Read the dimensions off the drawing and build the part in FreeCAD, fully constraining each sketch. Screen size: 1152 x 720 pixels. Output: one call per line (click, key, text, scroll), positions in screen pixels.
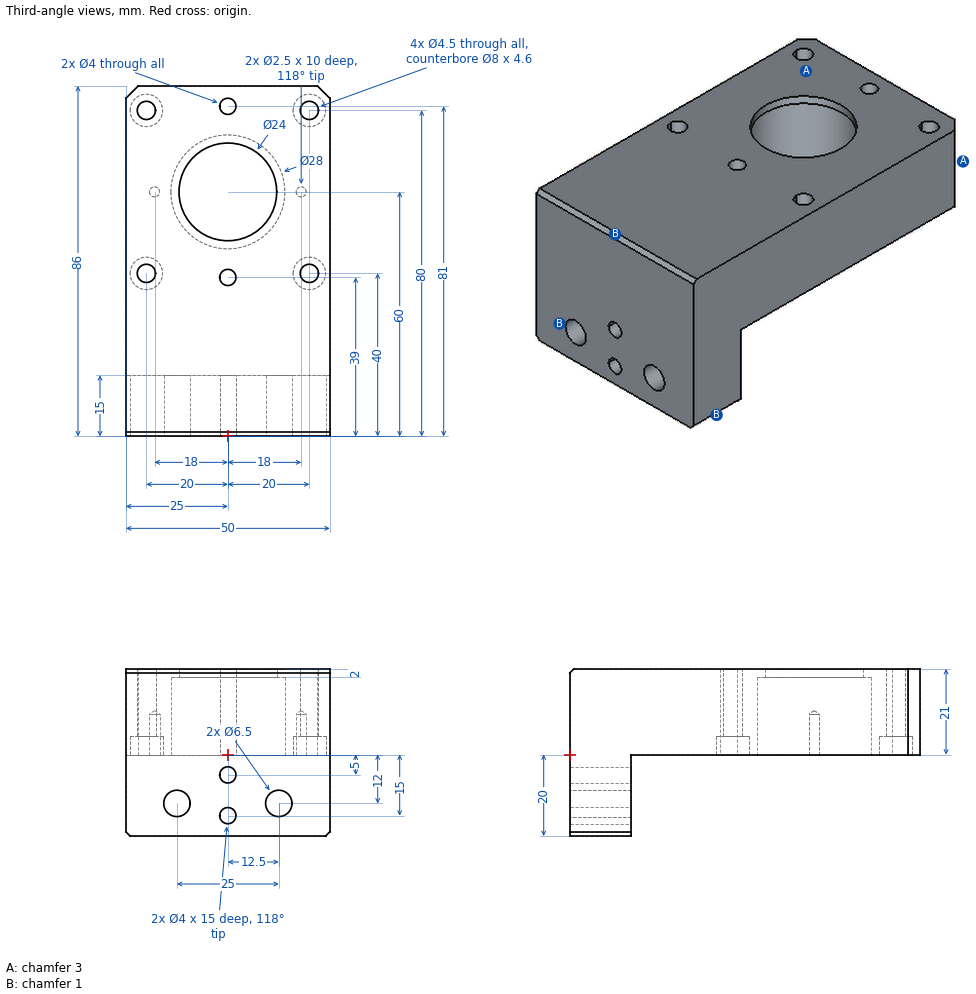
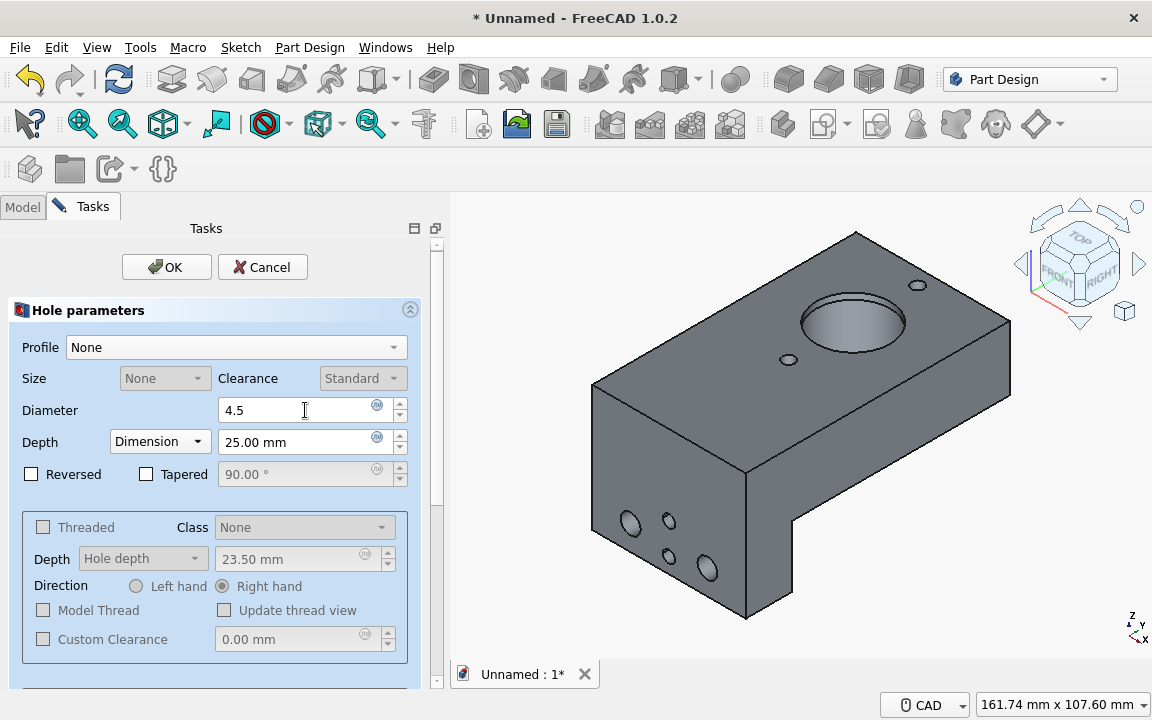
click(161, 442)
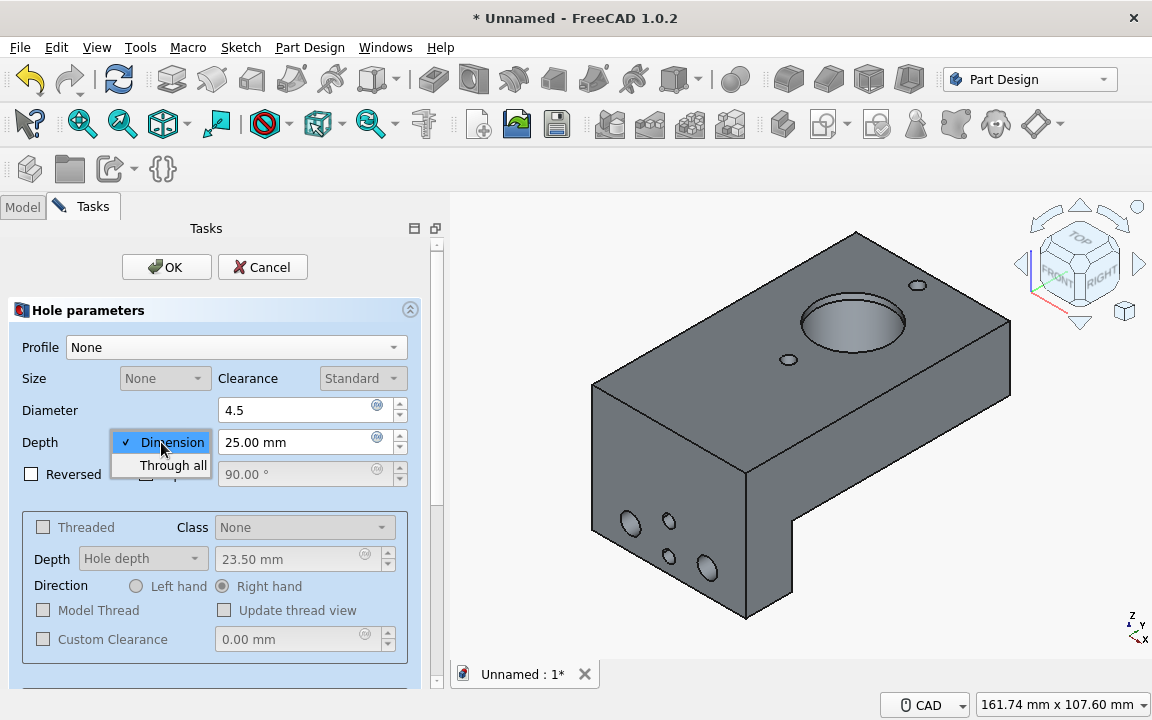
click(160, 466)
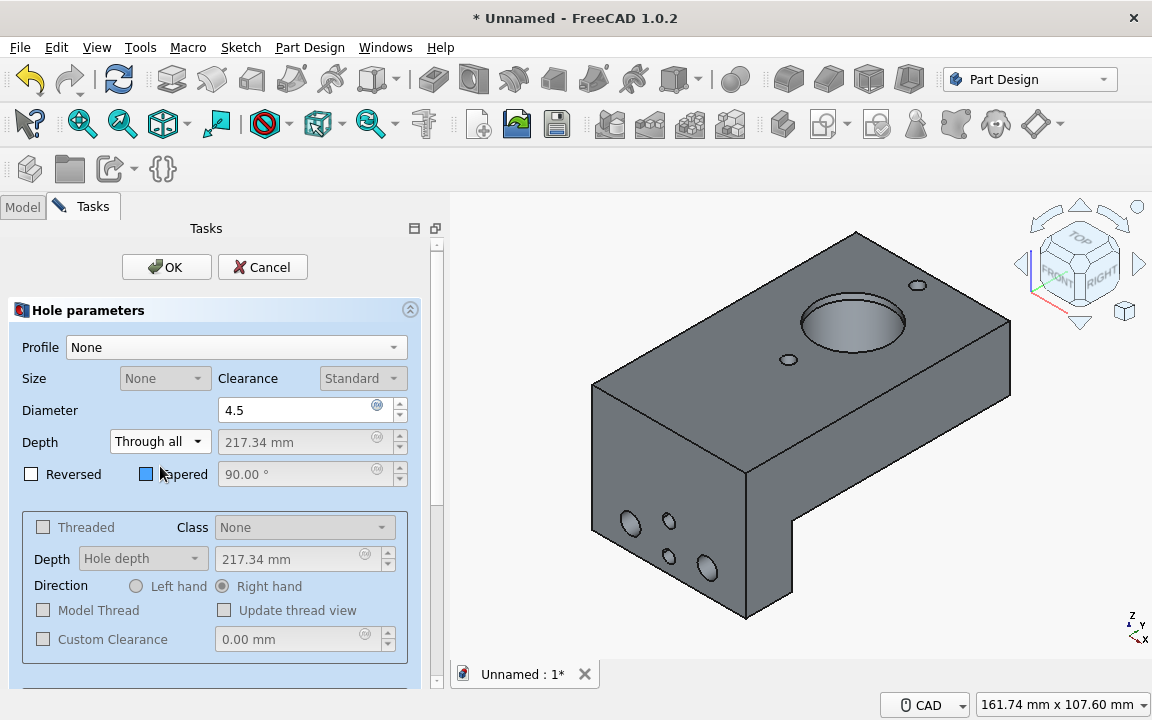
click(30, 474)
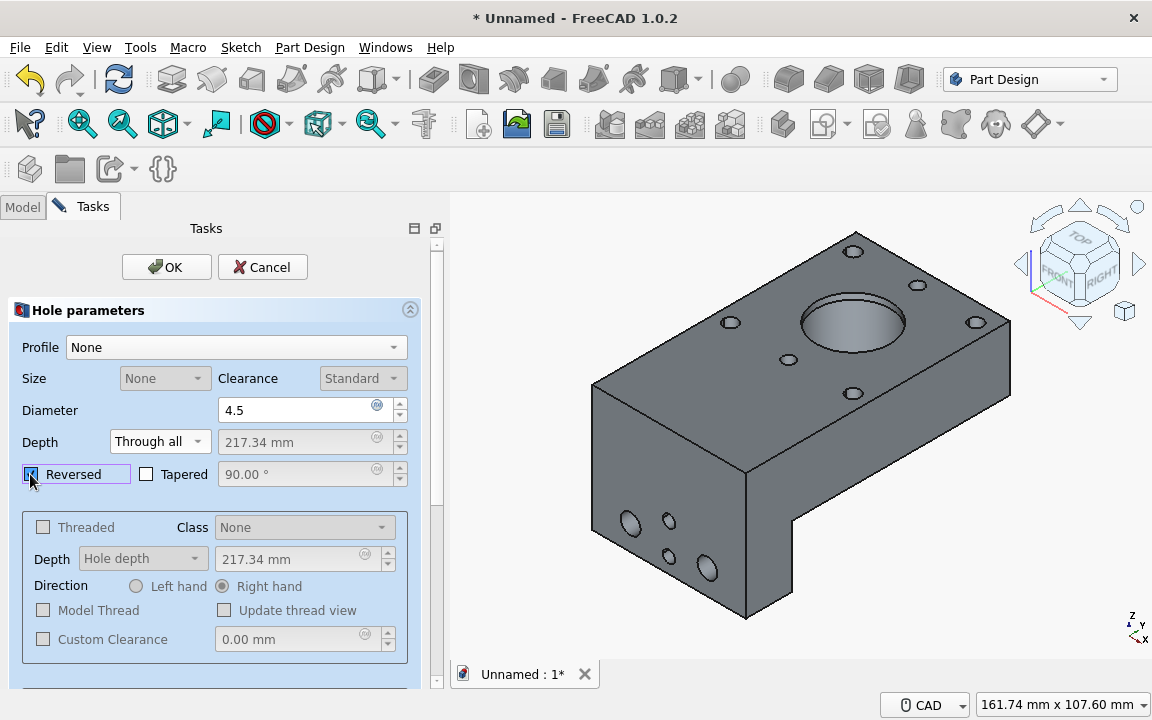
scroll(437, 463, down, 2)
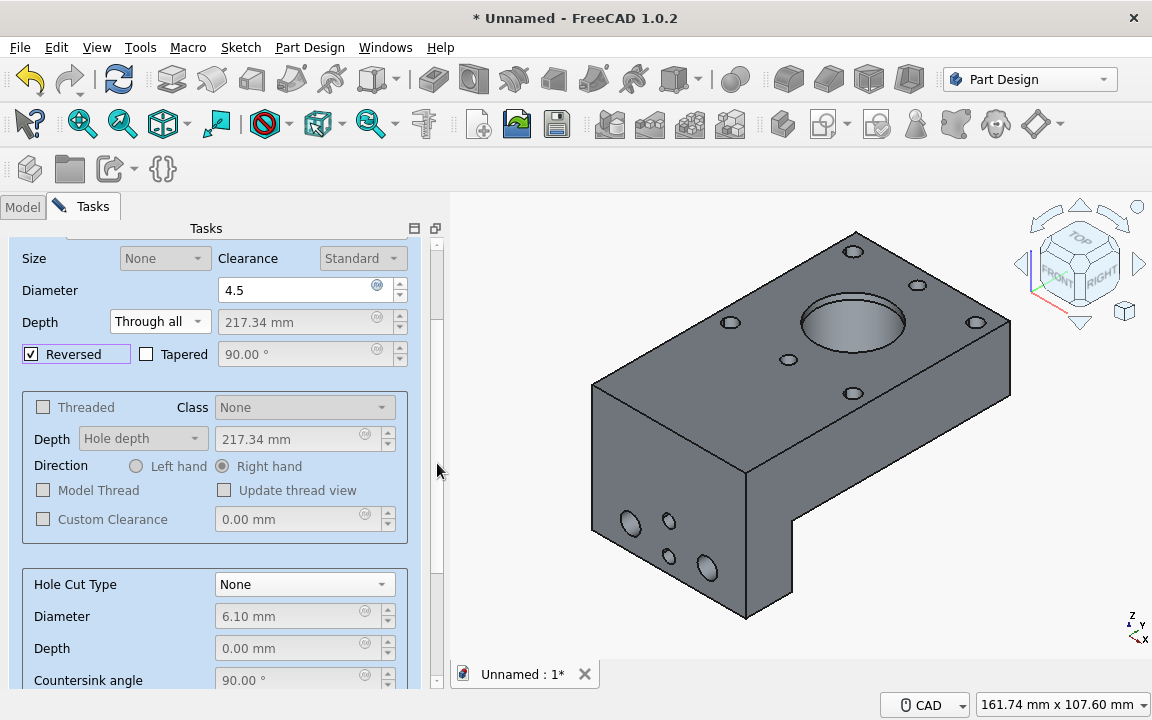
click(306, 584)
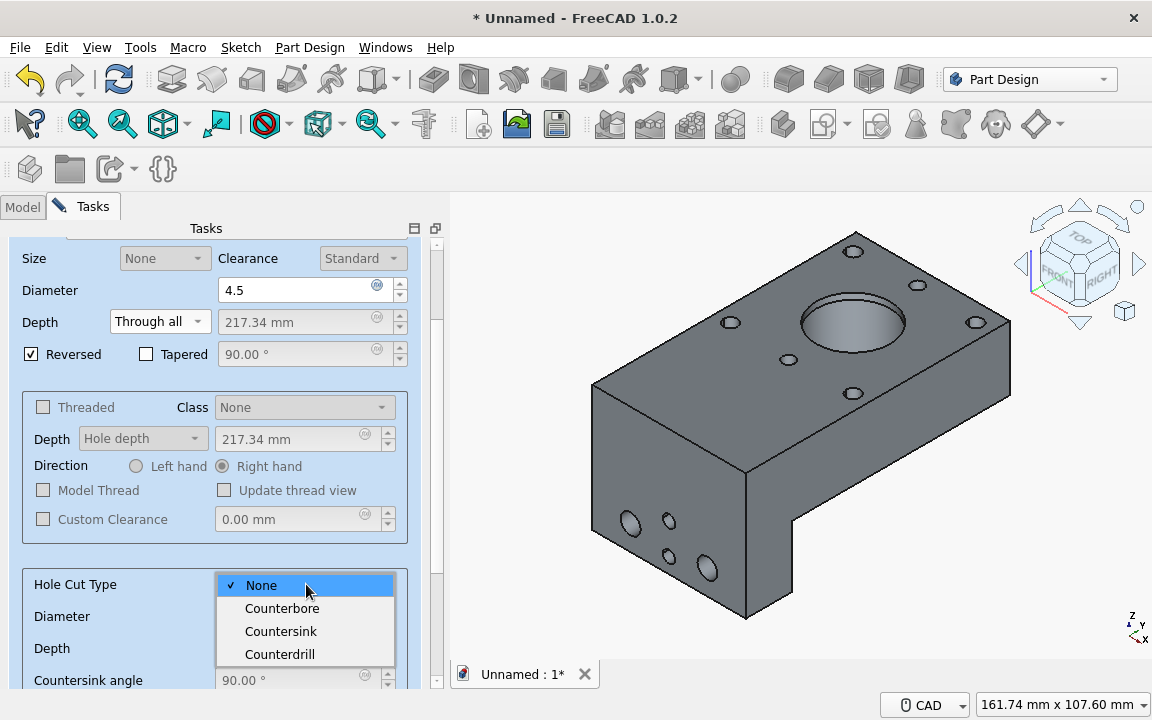
click(304, 608)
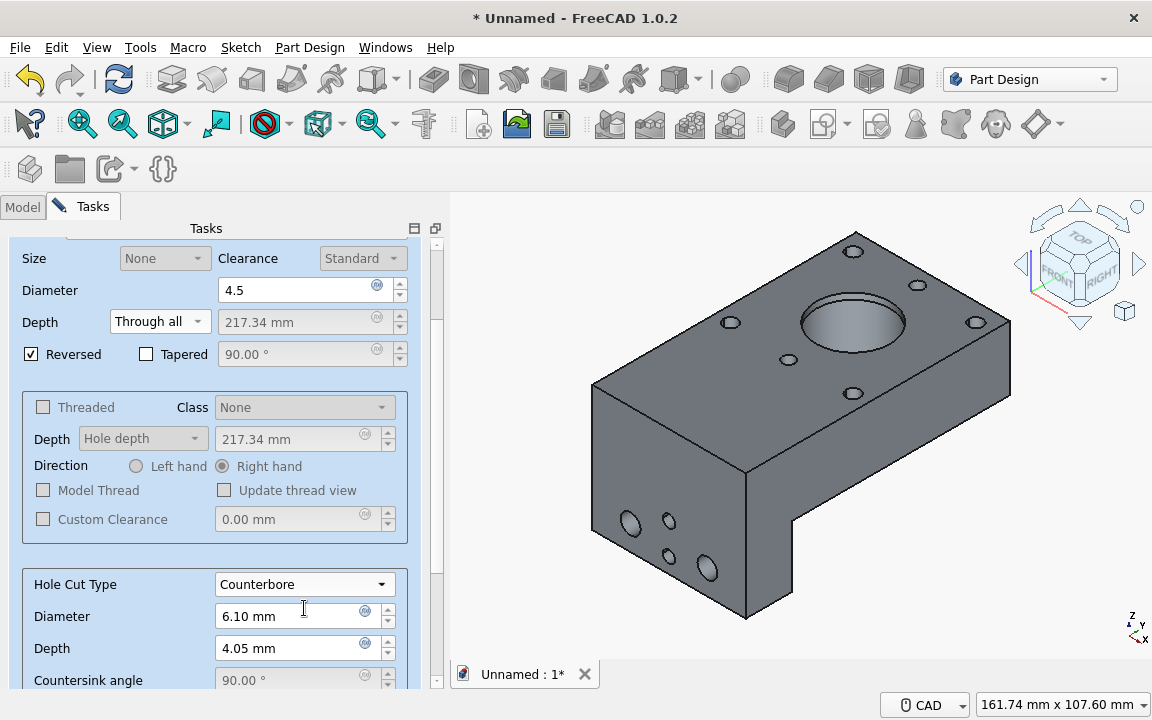
triple_click(298, 616)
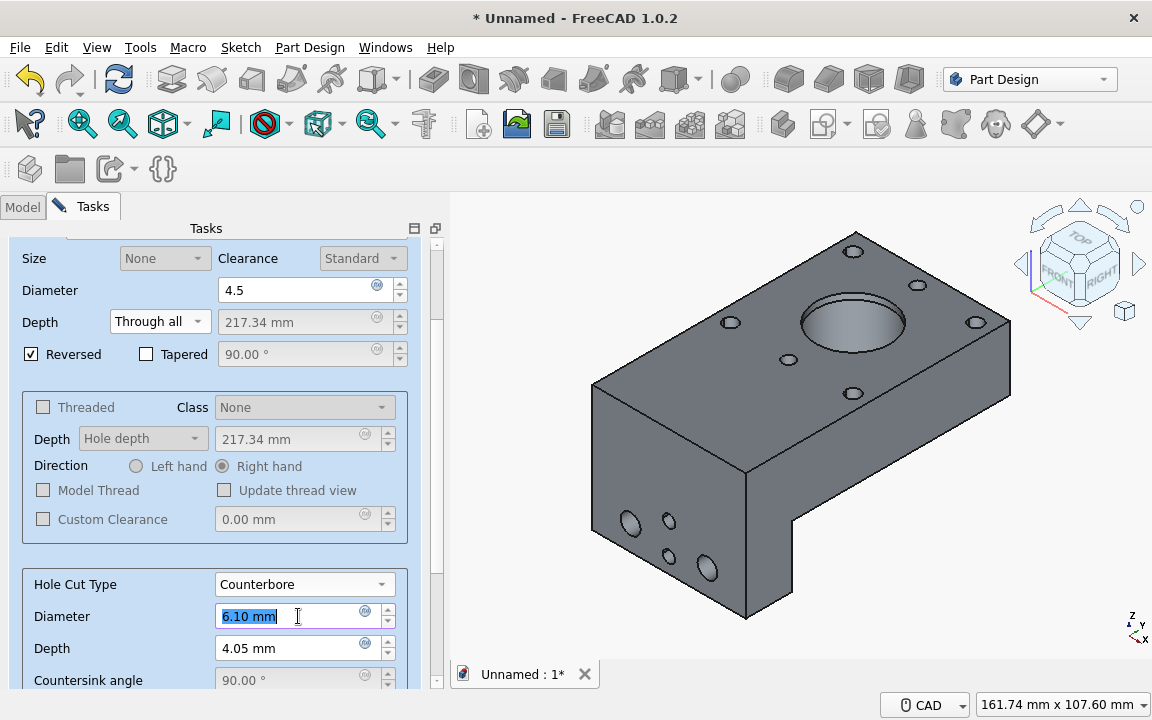
text(8)
key(Tab)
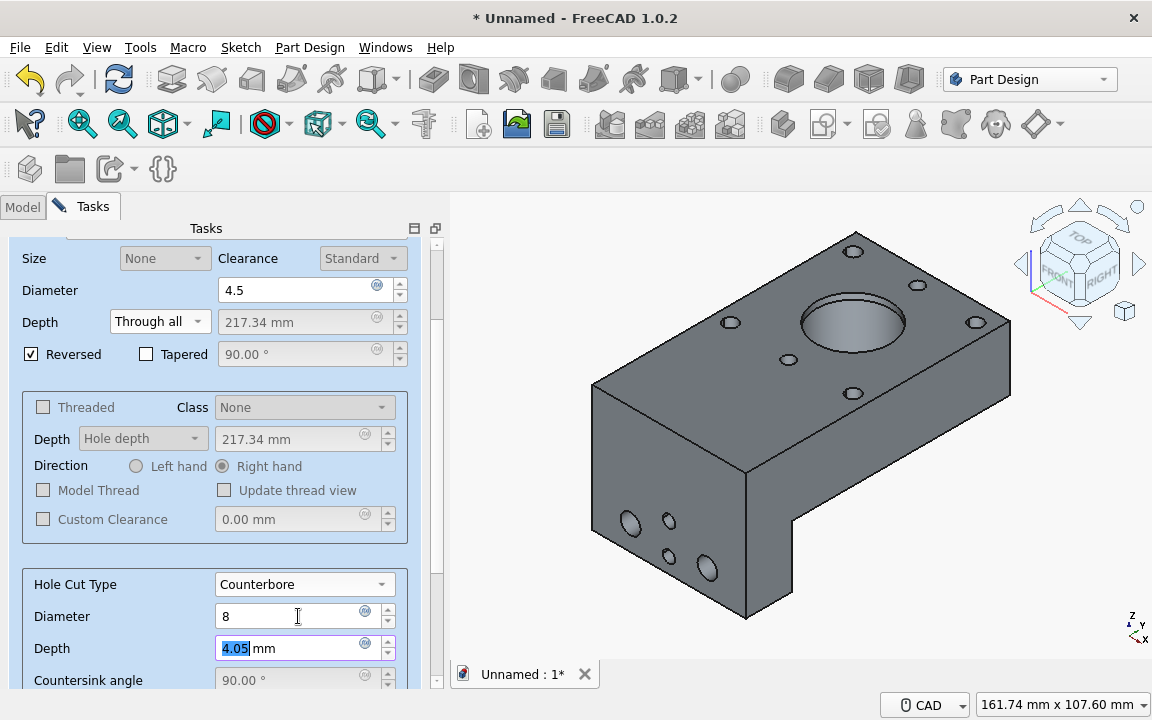
text(4.6)
key(Tab)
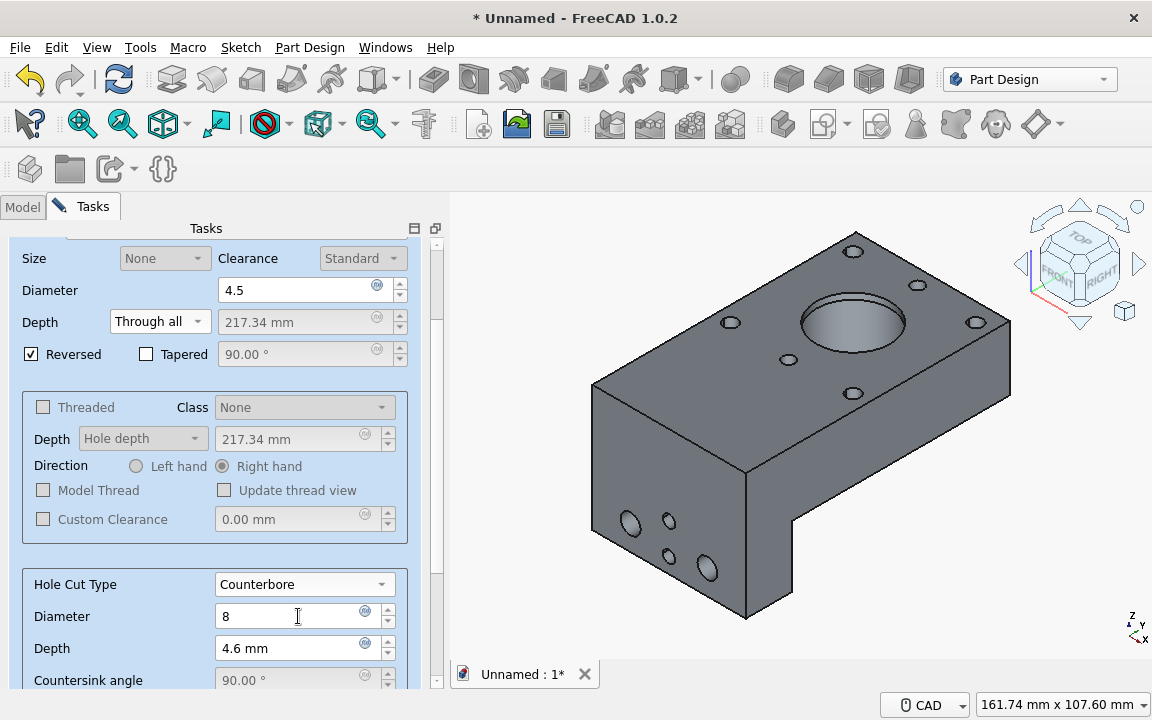
scroll(437, 463, up, 3)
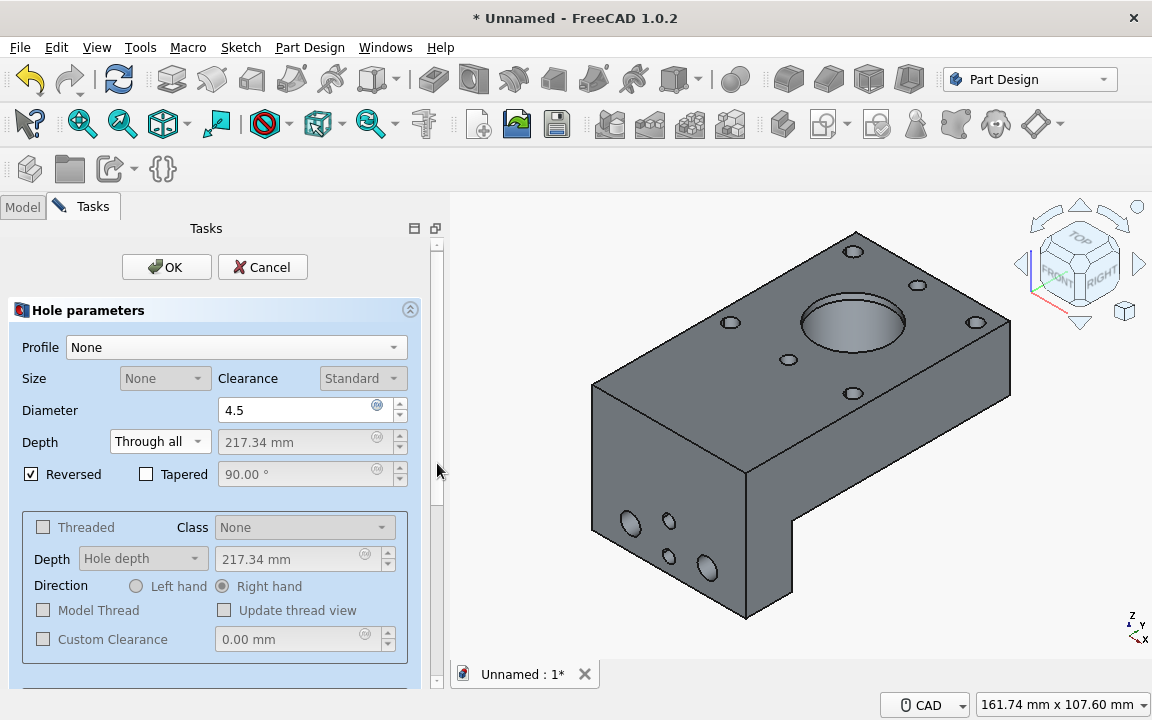
click(167, 267)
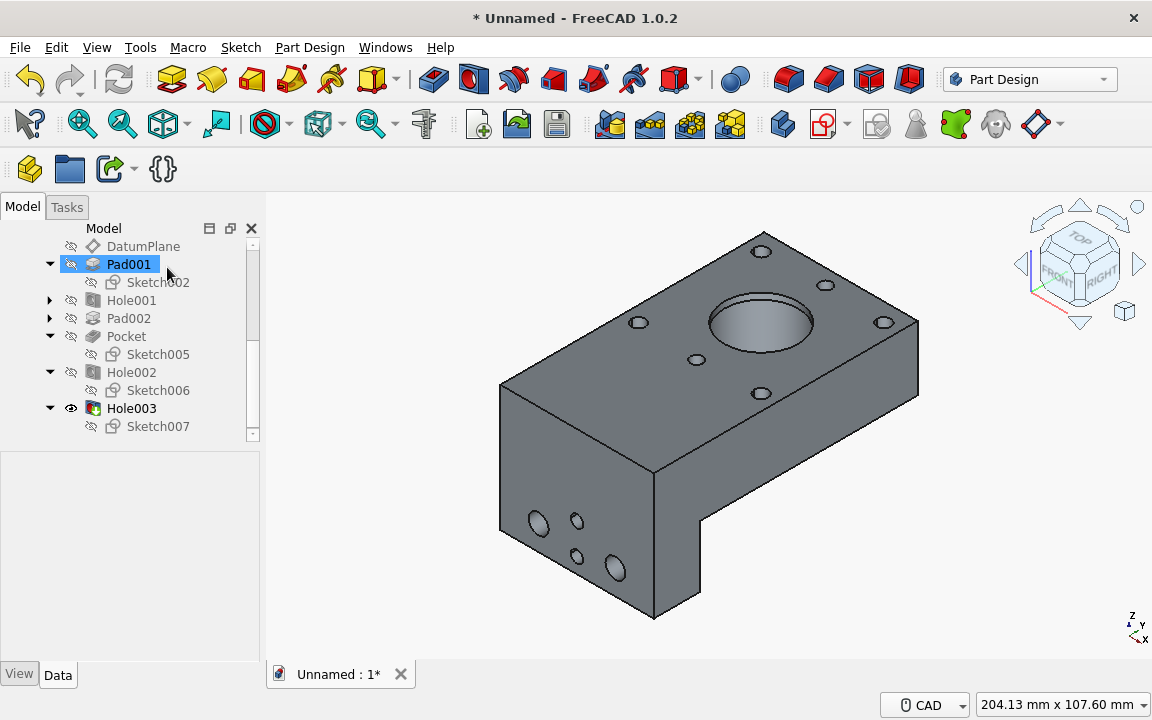
key(2)